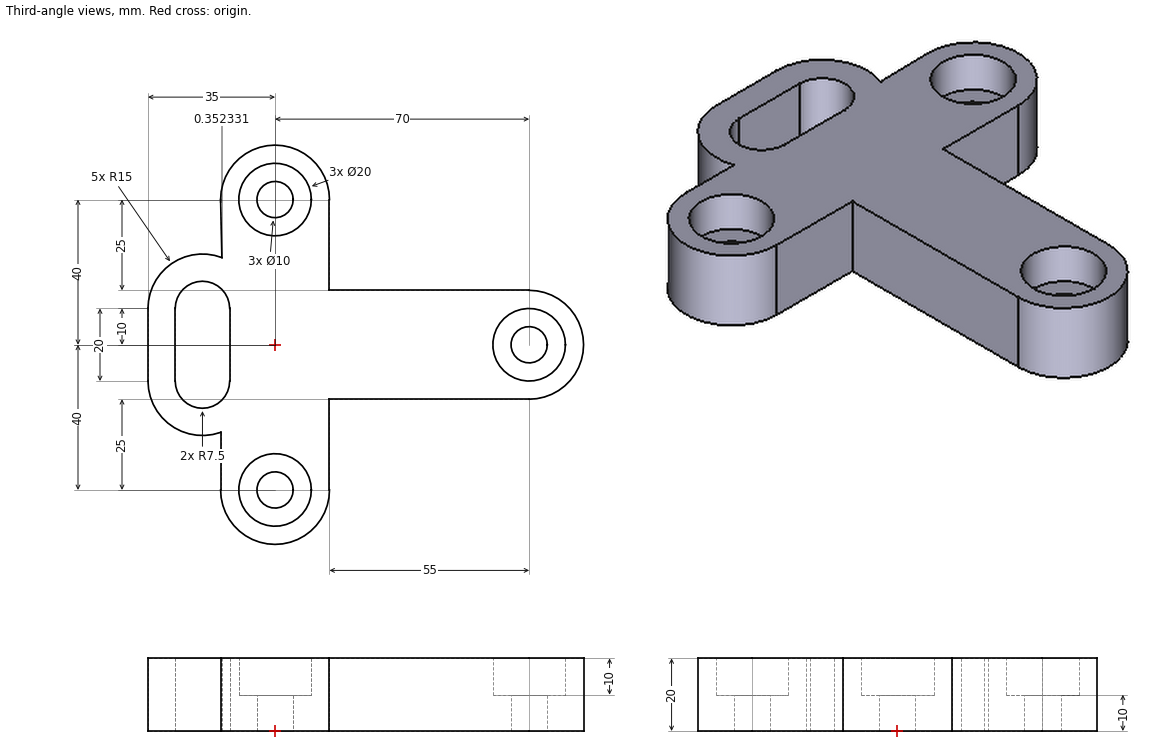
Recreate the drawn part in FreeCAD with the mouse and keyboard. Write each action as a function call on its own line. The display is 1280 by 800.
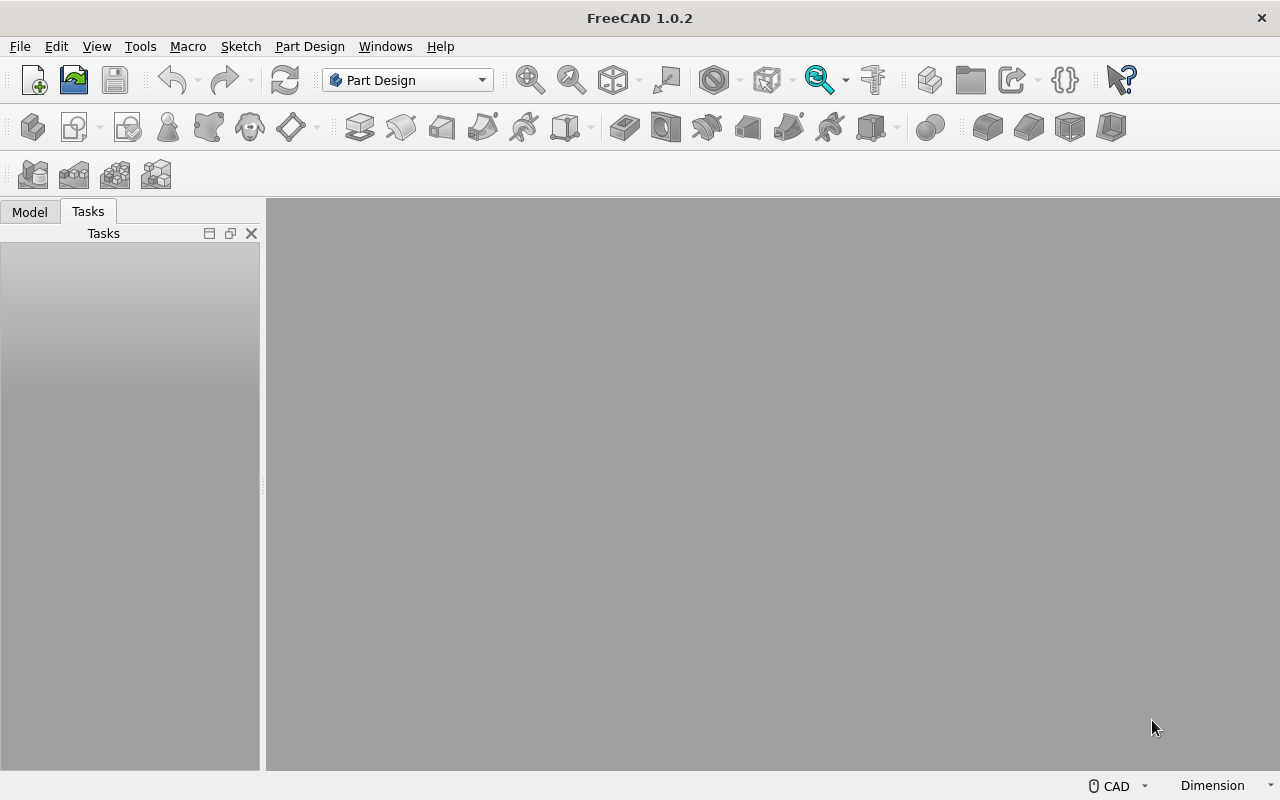
click(33, 80)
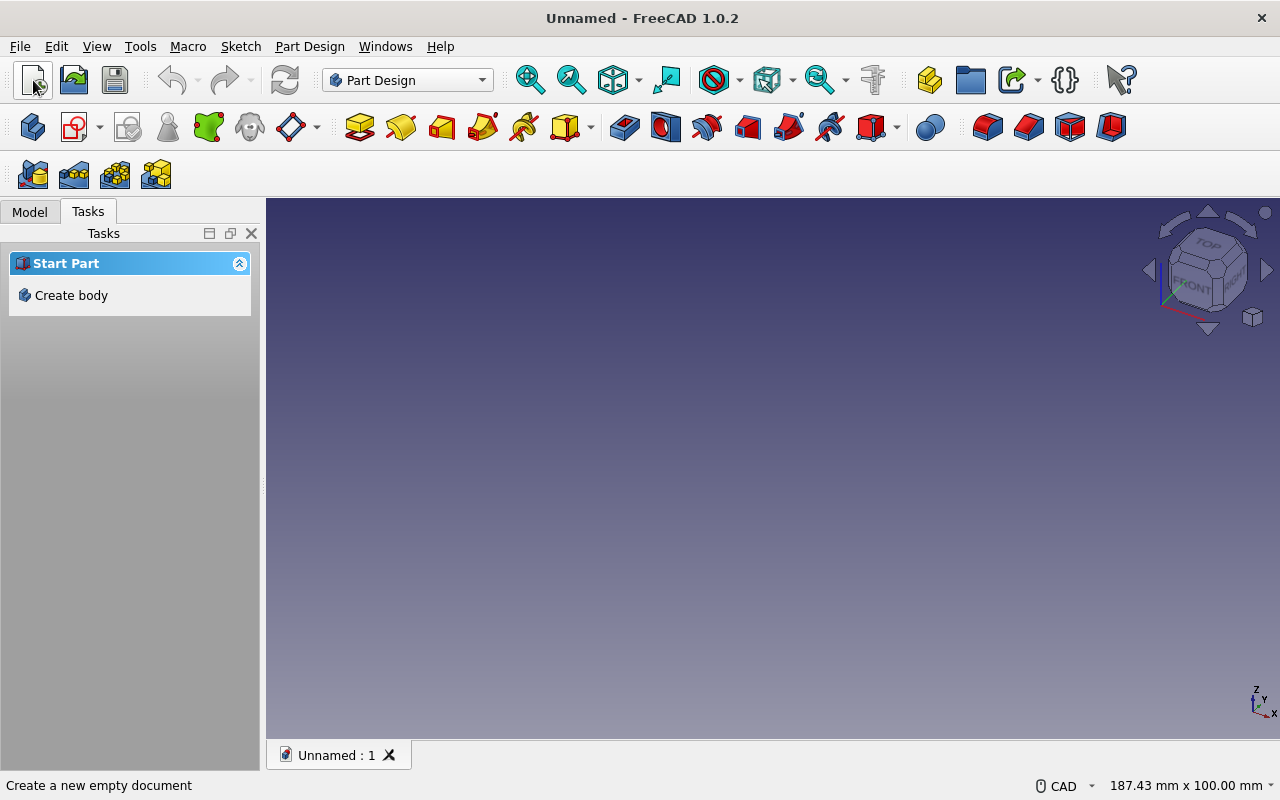
click(74, 128)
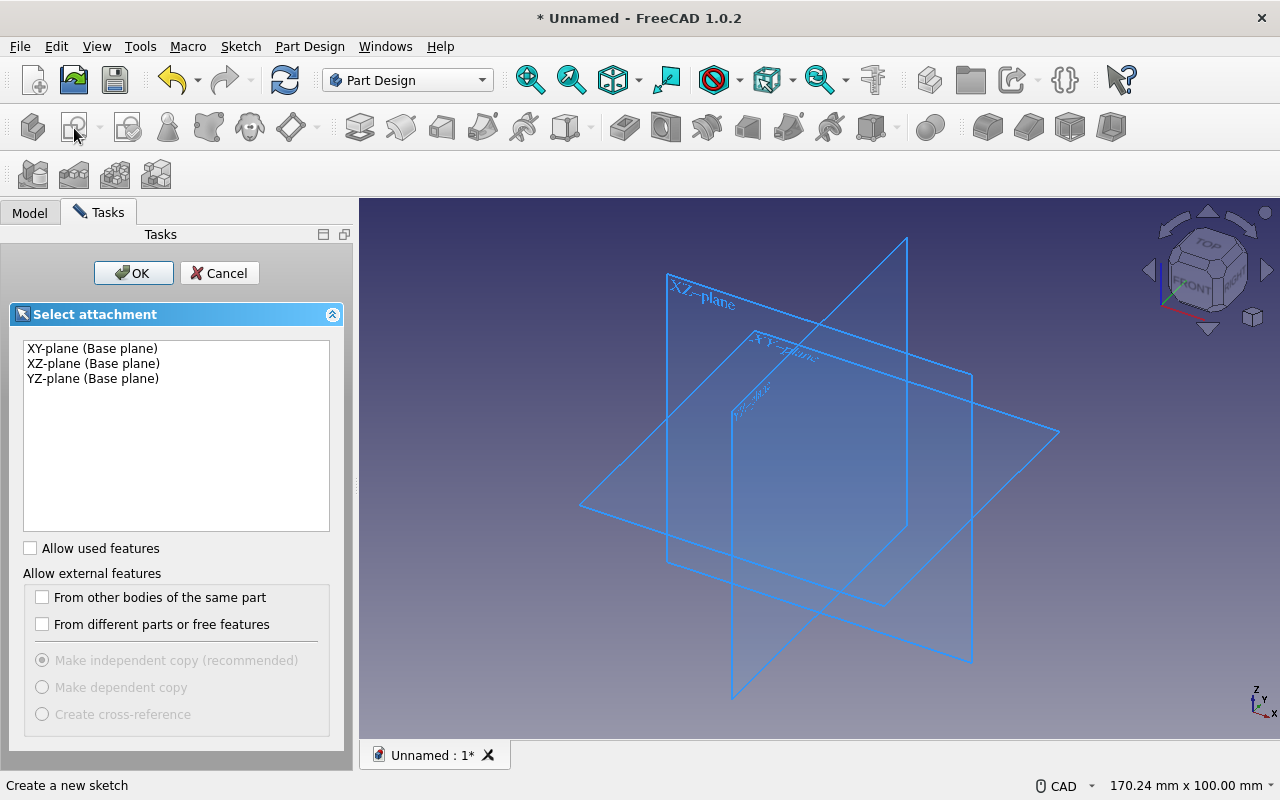
click(84, 348)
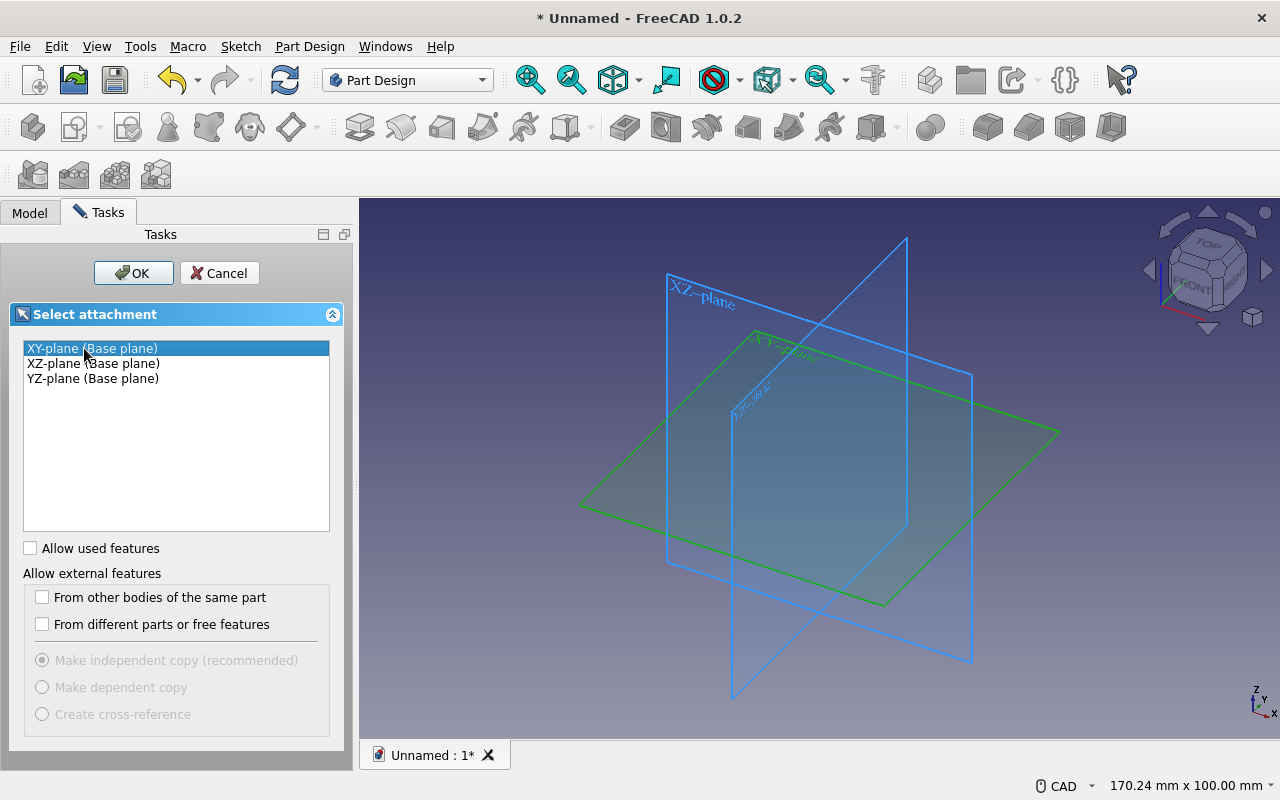
click(134, 273)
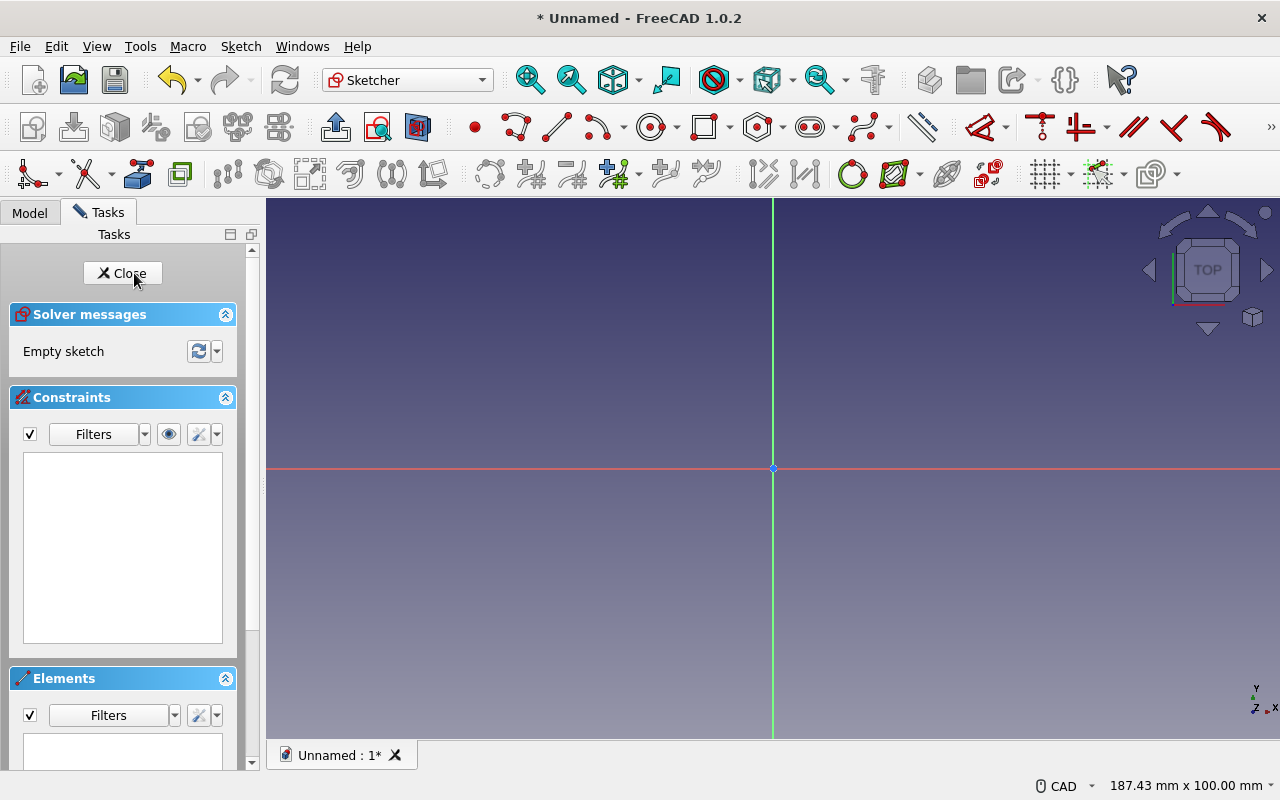
scroll(457, 468, down, 3)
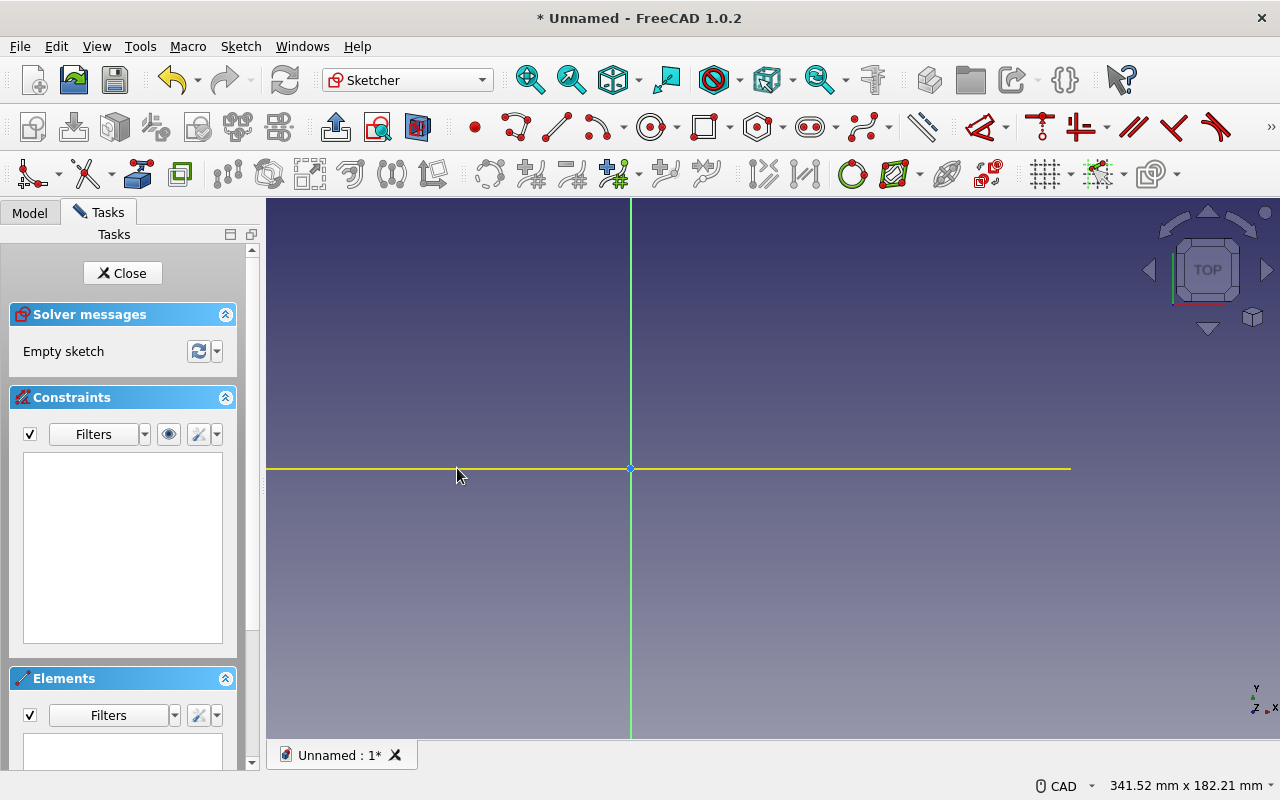
click(557, 128)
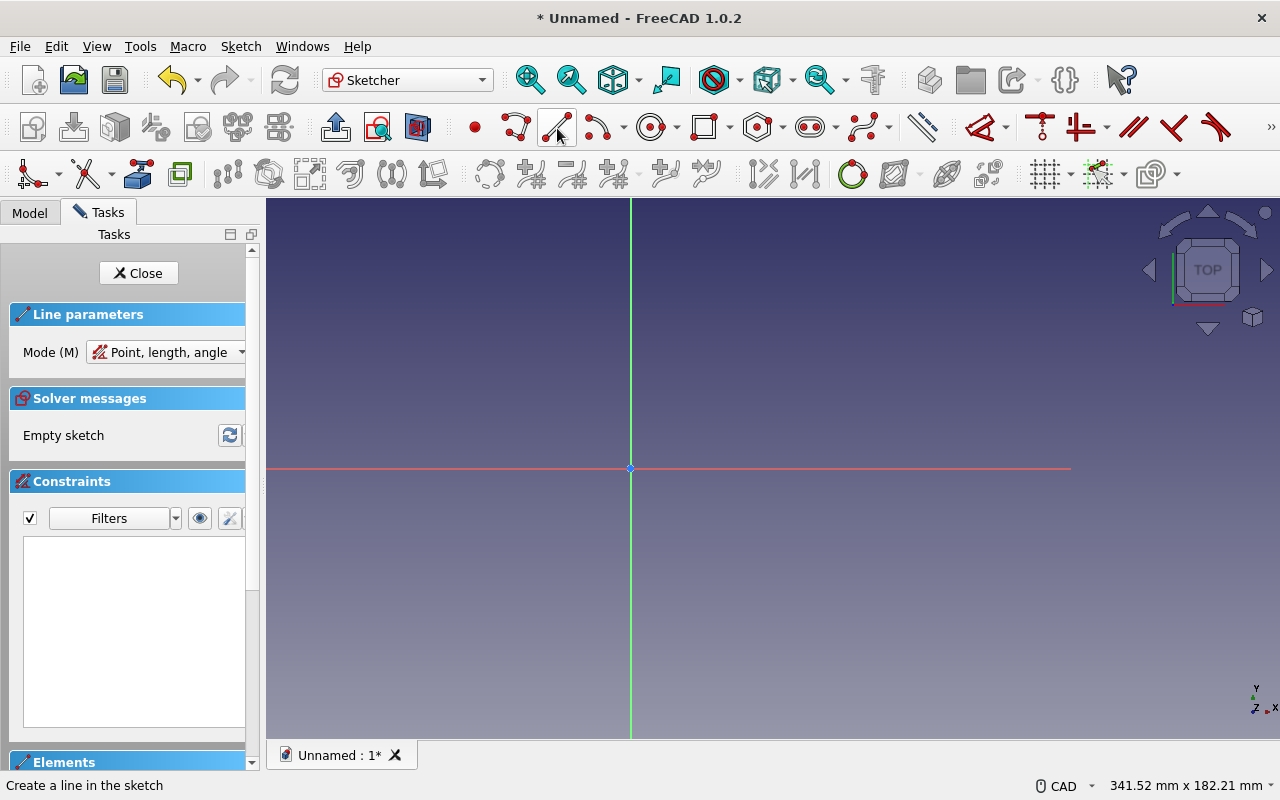
click(527, 439)
click(527, 498)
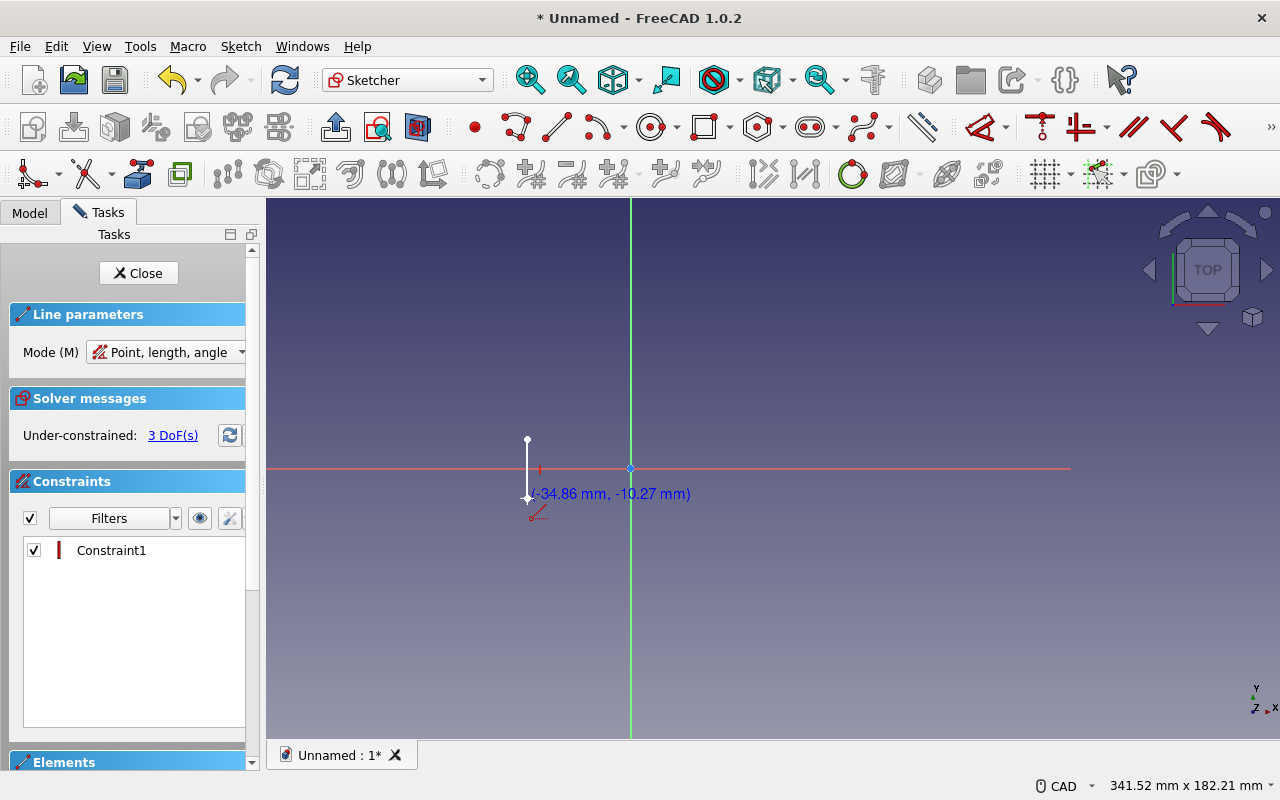
click(586, 540)
click(586, 587)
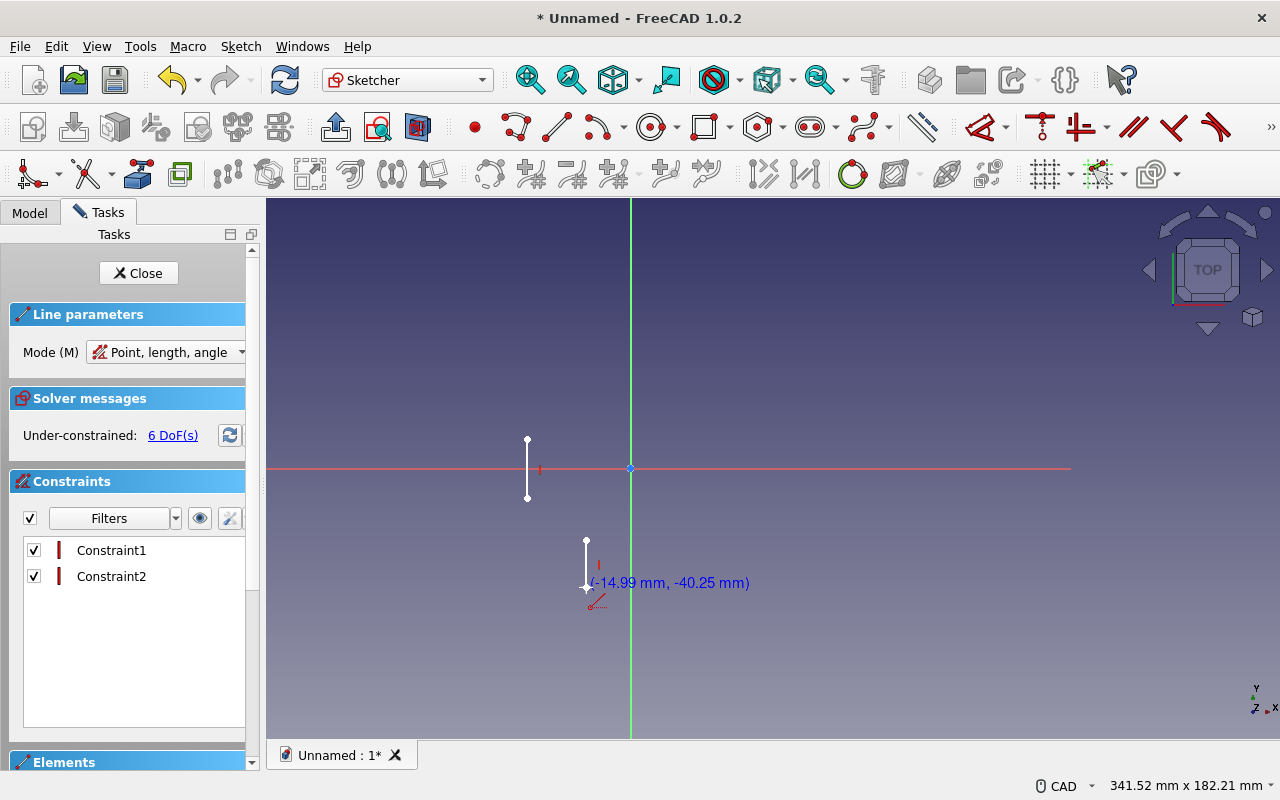
click(516, 128)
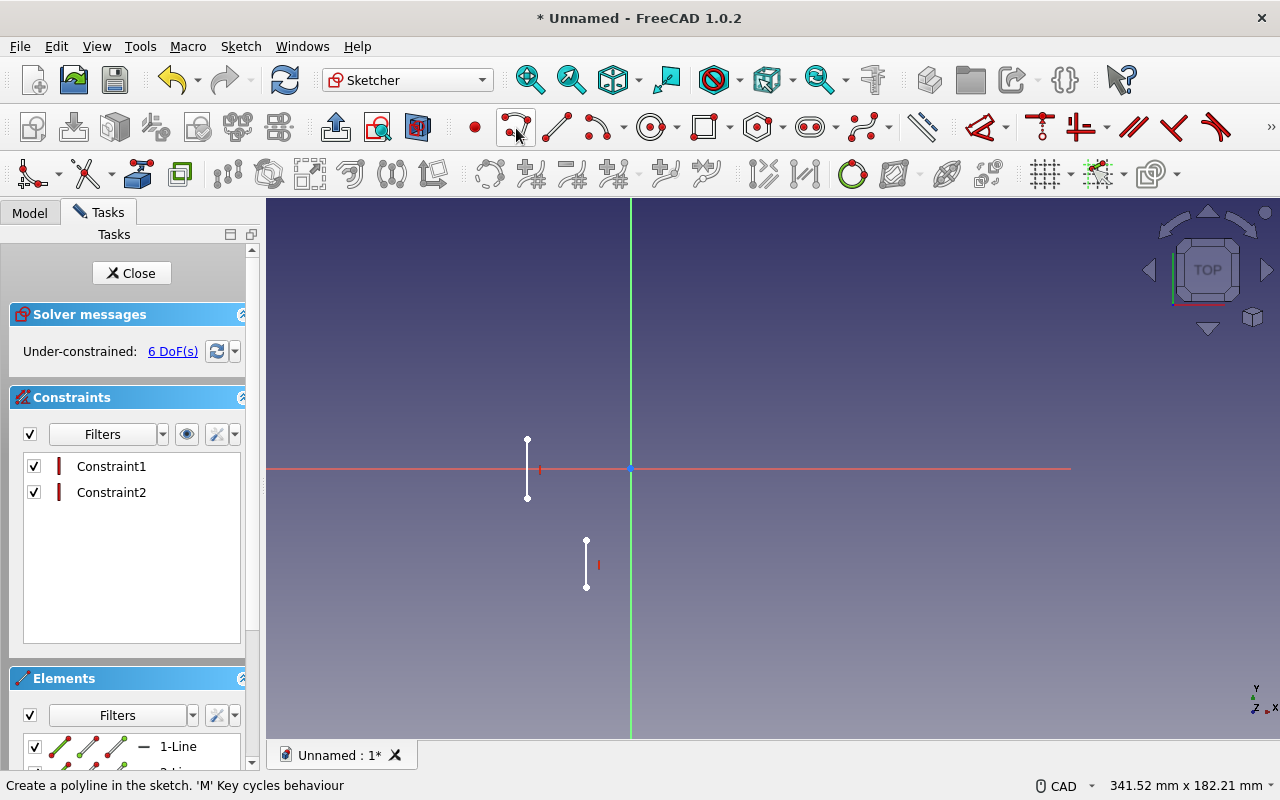
click(675, 587)
click(675, 513)
click(838, 513)
right_click(838, 513)